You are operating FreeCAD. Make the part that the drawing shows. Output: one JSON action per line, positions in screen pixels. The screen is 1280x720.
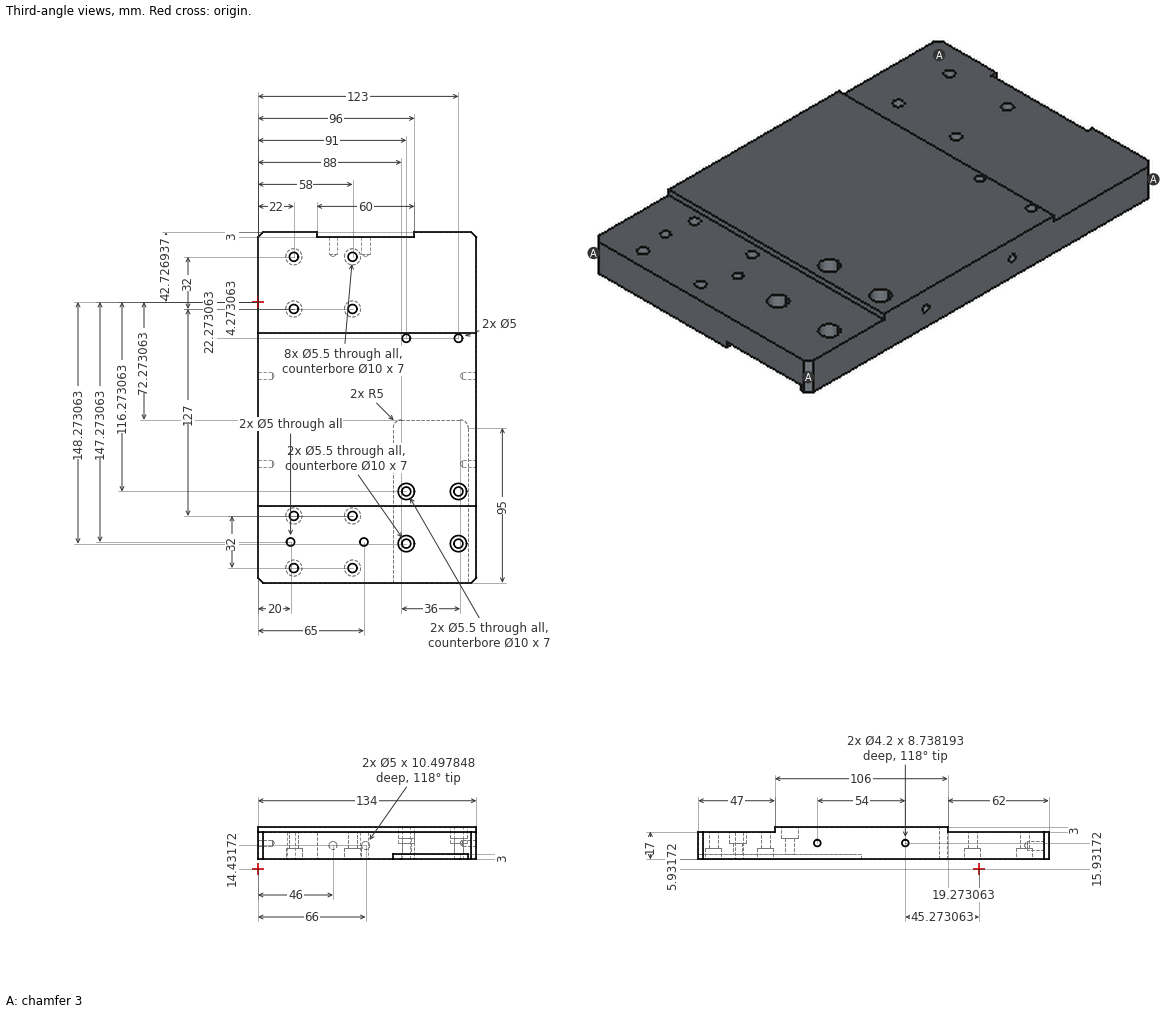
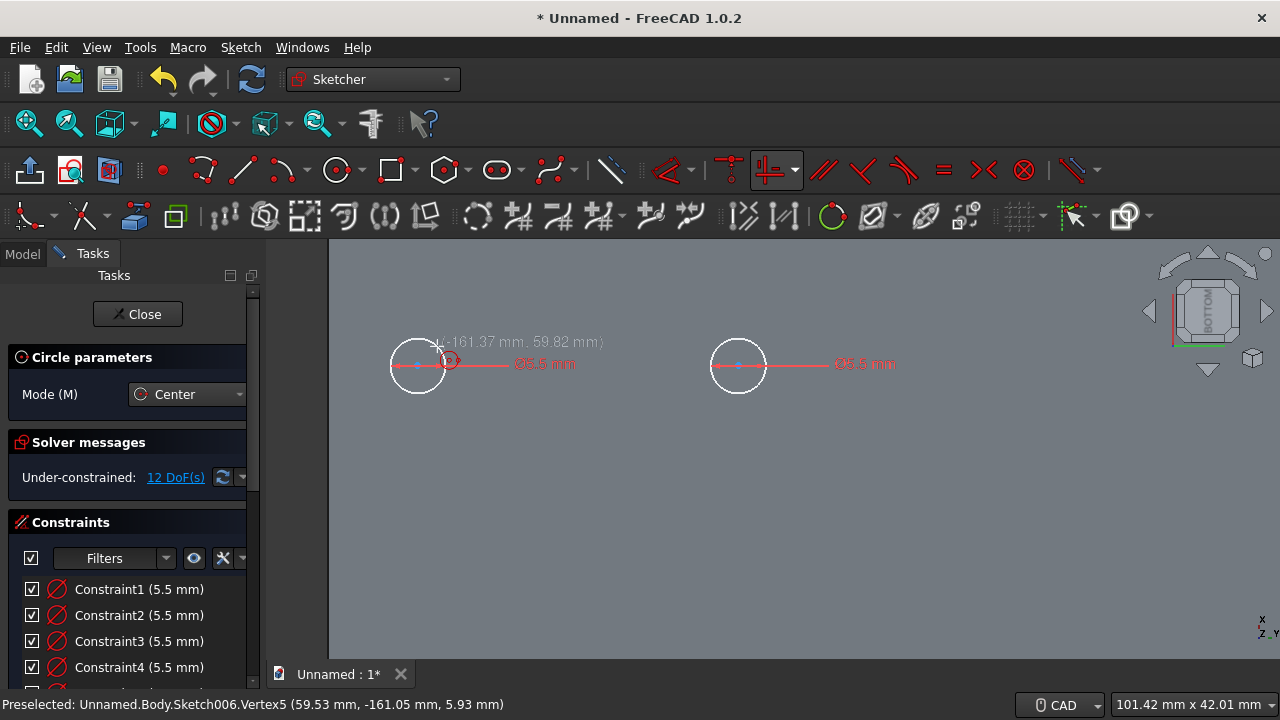
{"action": "scroll", "coordinate": [416, 366], "scroll_direction": "down", "scroll_amount": 6}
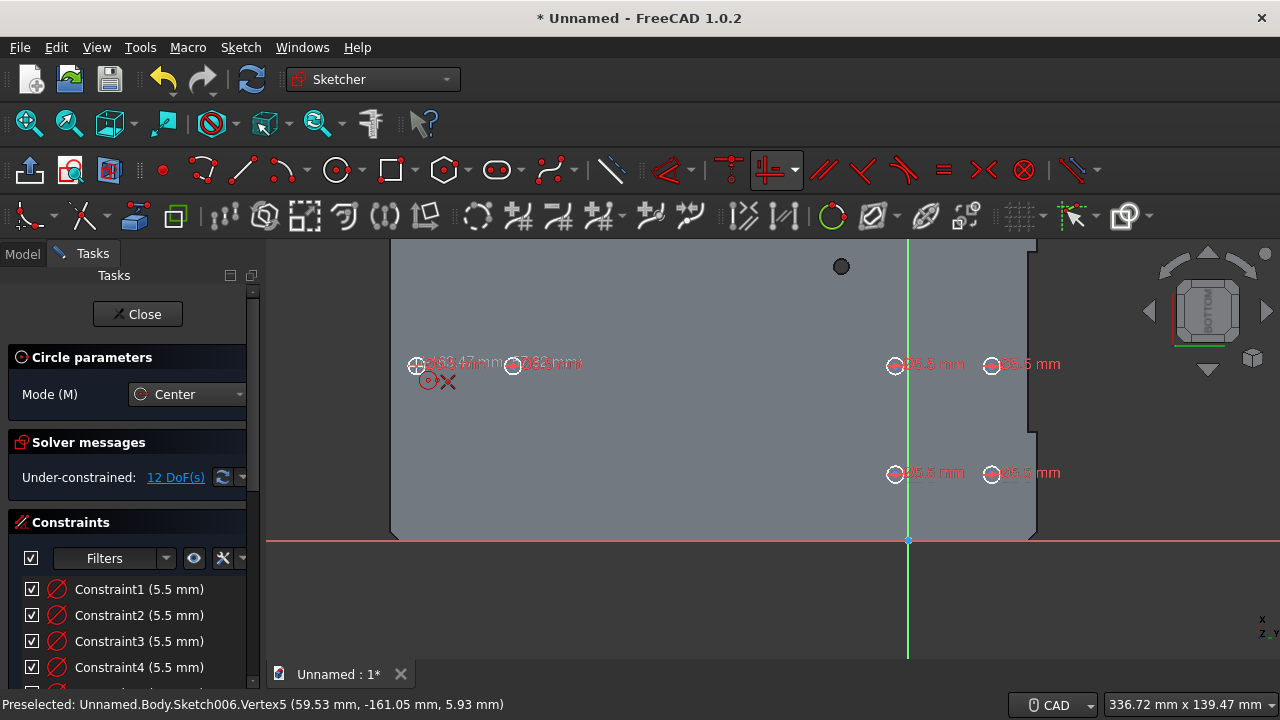
{"action": "scroll", "coordinate": [417, 474], "scroll_direction": "up", "scroll_amount": 6}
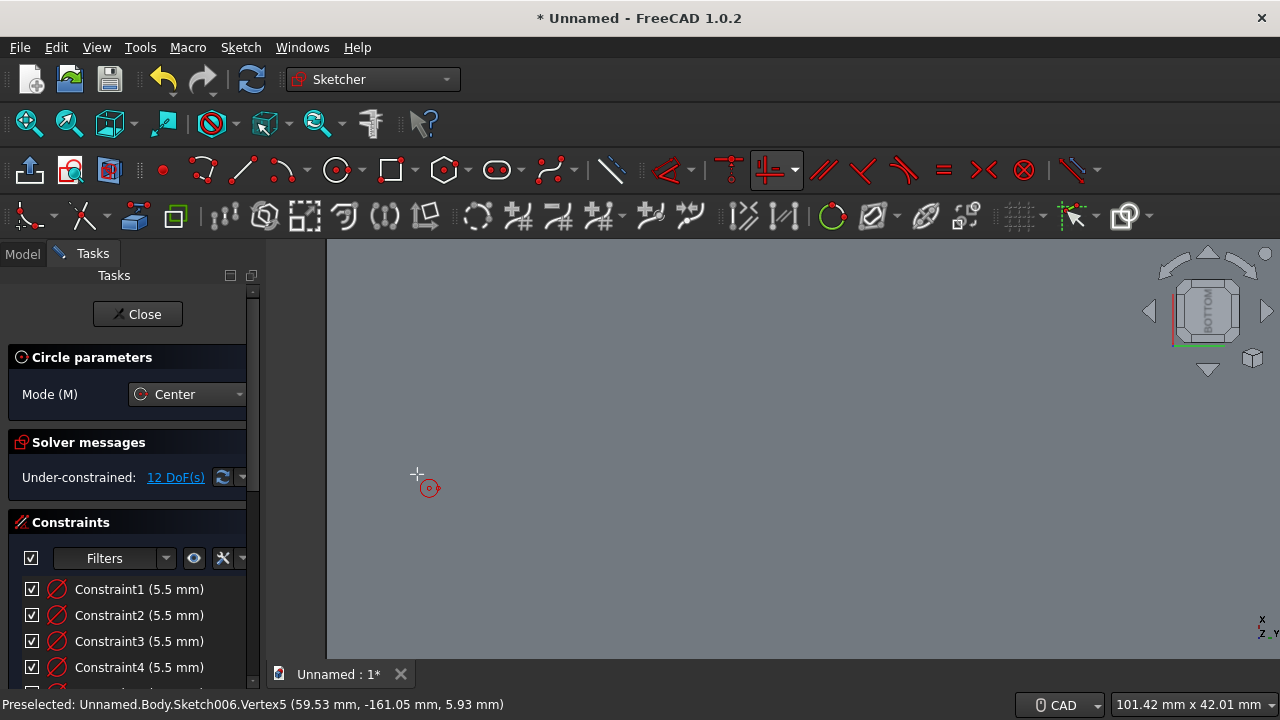
{"action": "left_click", "coordinate": [416, 474]}
{"action": "mouse_move", "coordinate": [435, 455]}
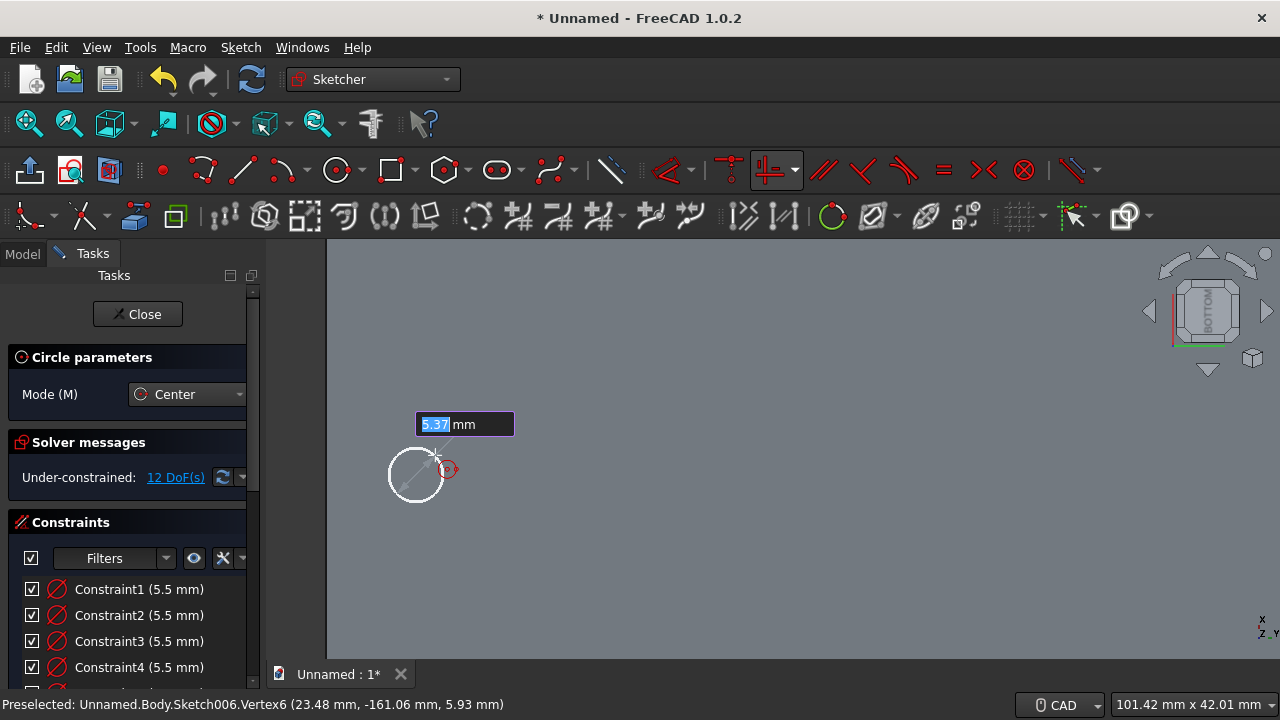
{"action": "type", "text": "5.5"}
{"action": "key", "text": "Return"}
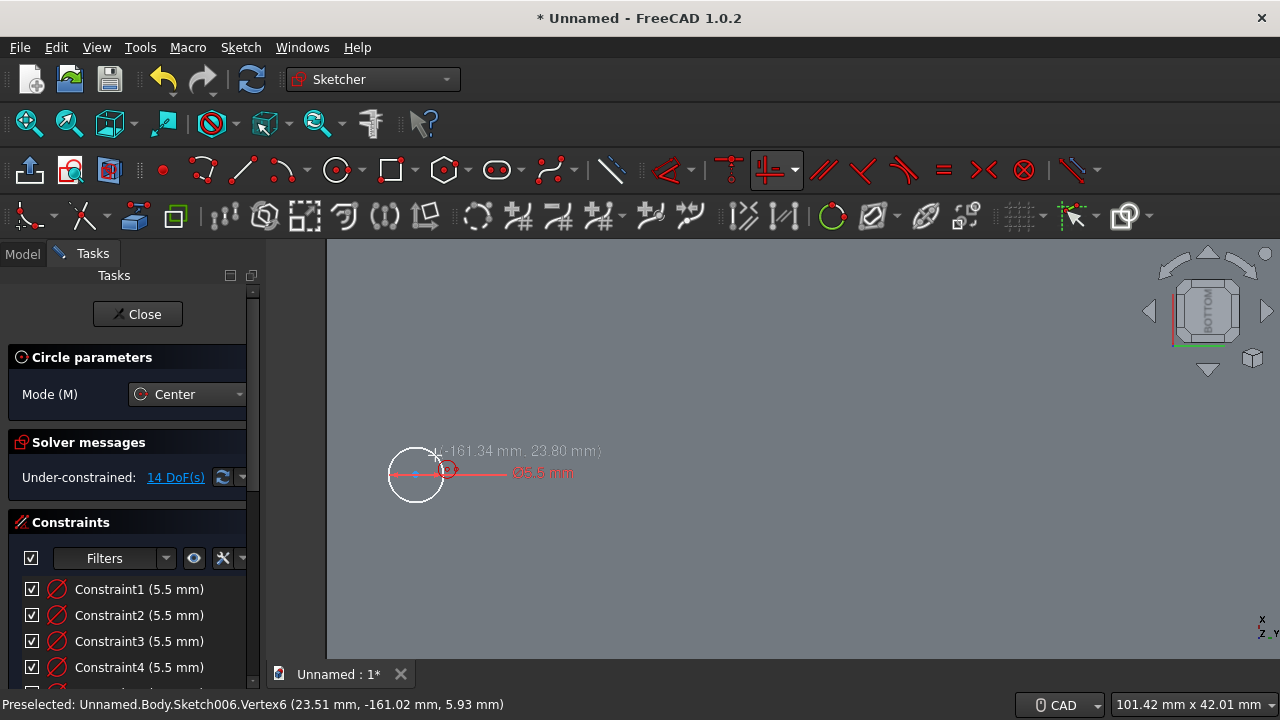
{"action": "left_click", "coordinate": [736, 474]}
{"action": "mouse_move", "coordinate": [755, 455]}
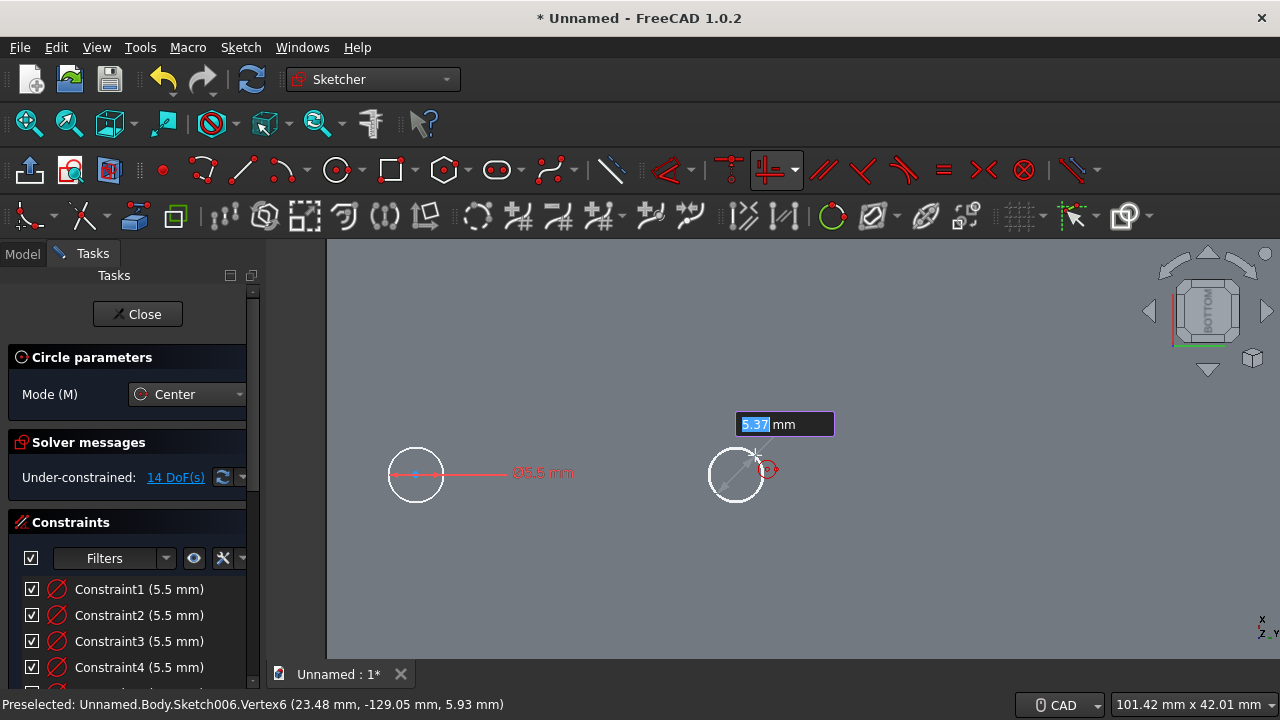
{"action": "type", "text": "5.5"}
{"action": "key", "text": "Return"}
{"action": "key", "text": "Escape"}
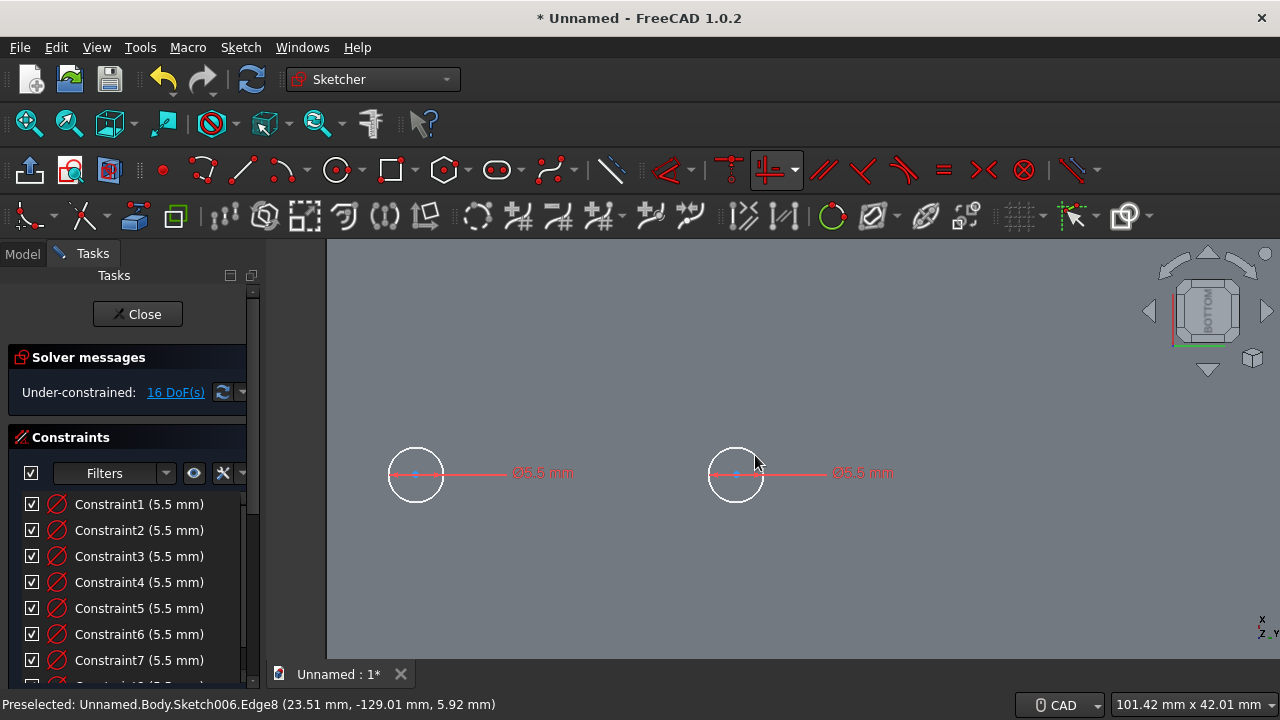
{"action": "scroll", "coordinate": [417, 474], "scroll_direction": "down", "scroll_amount": 6}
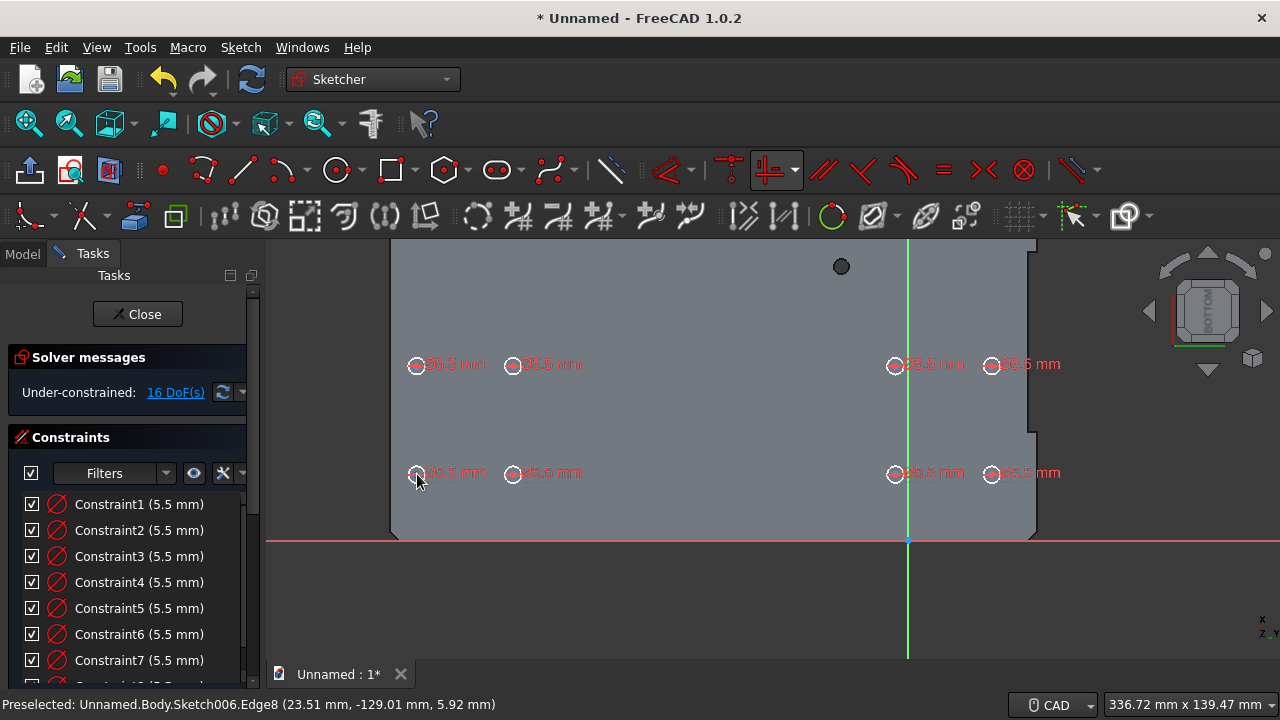
{"action": "left_click", "coordinate": [992, 366]}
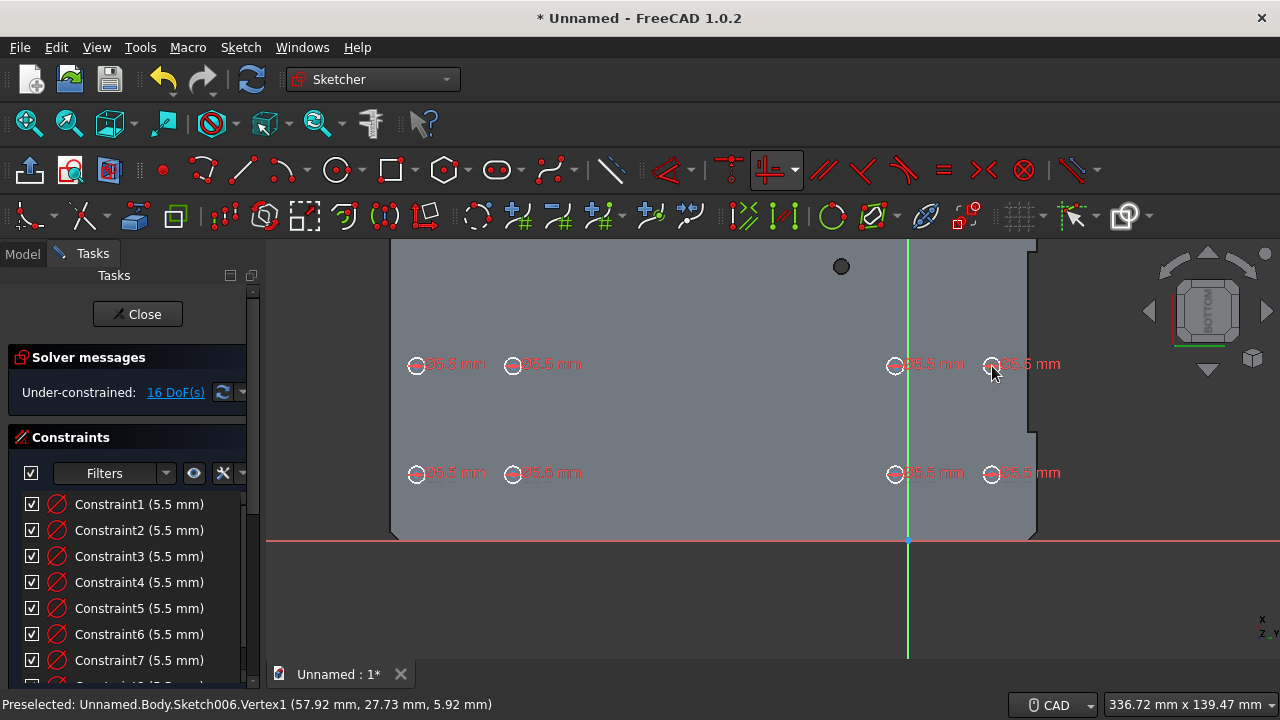
{"action": "left_click", "coordinate": [992, 475]}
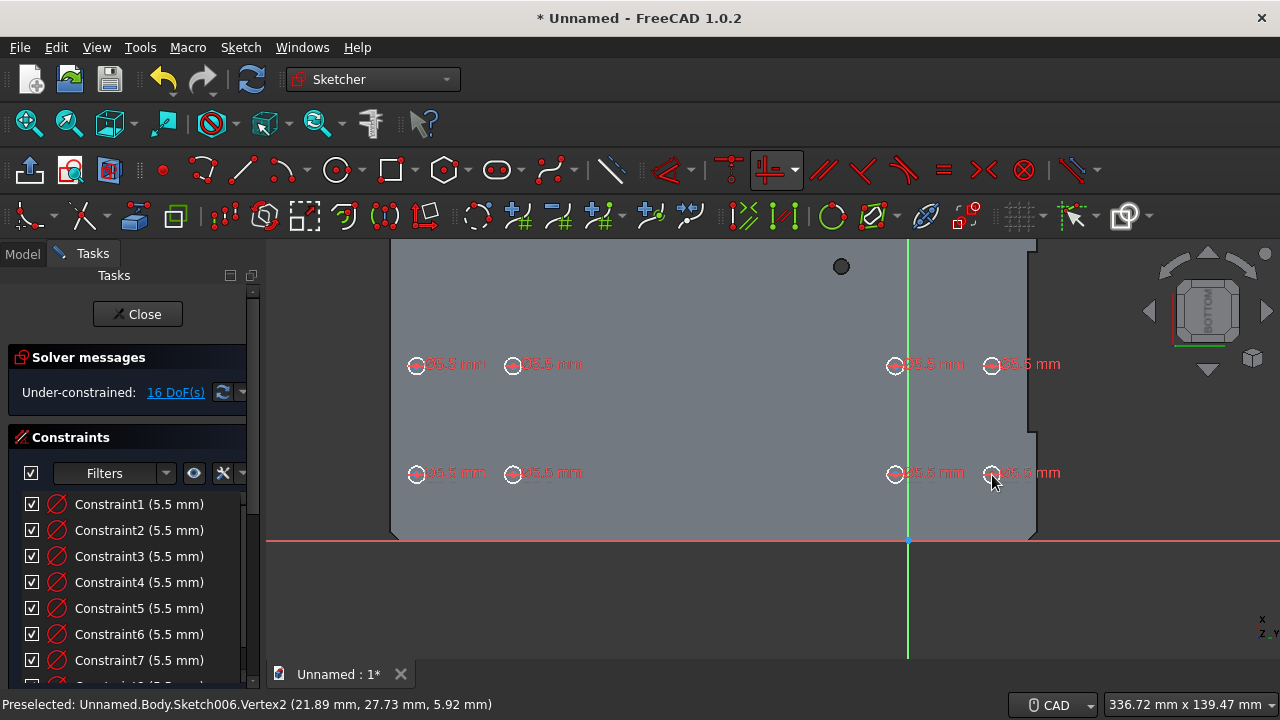
{"action": "left_click", "coordinate": [798, 170]}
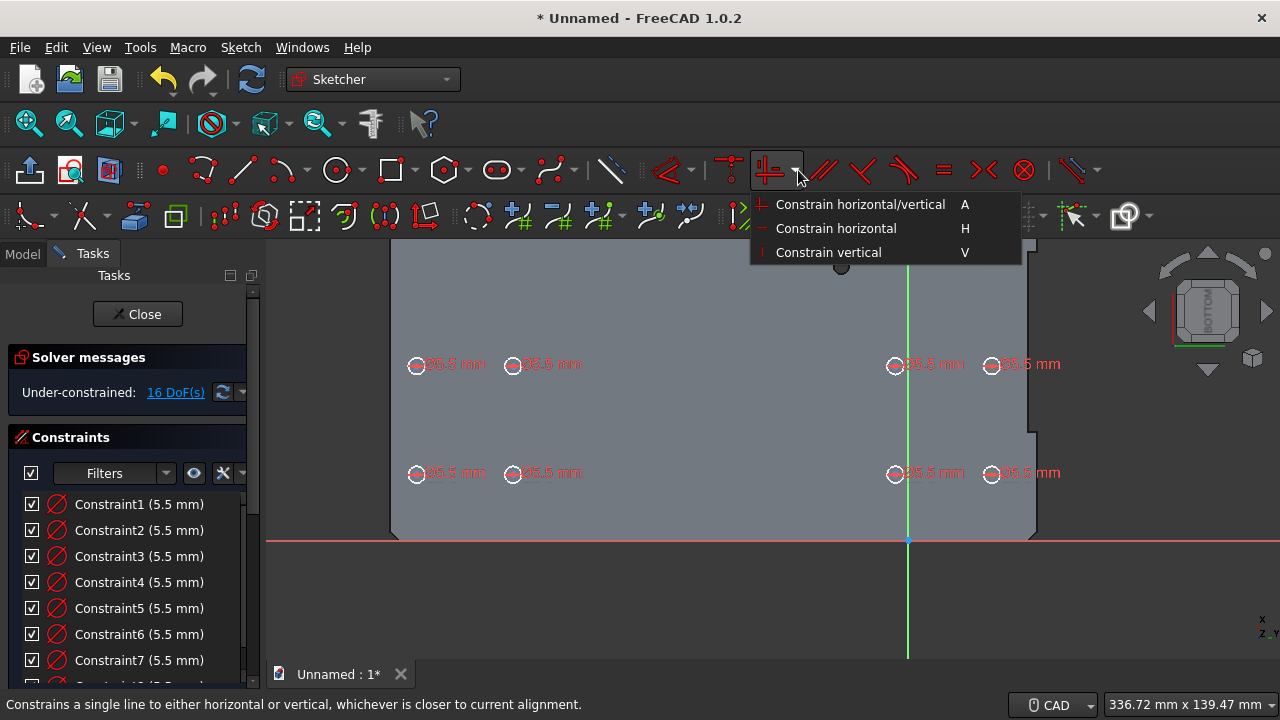
{"action": "left_click", "coordinate": [886, 252]}